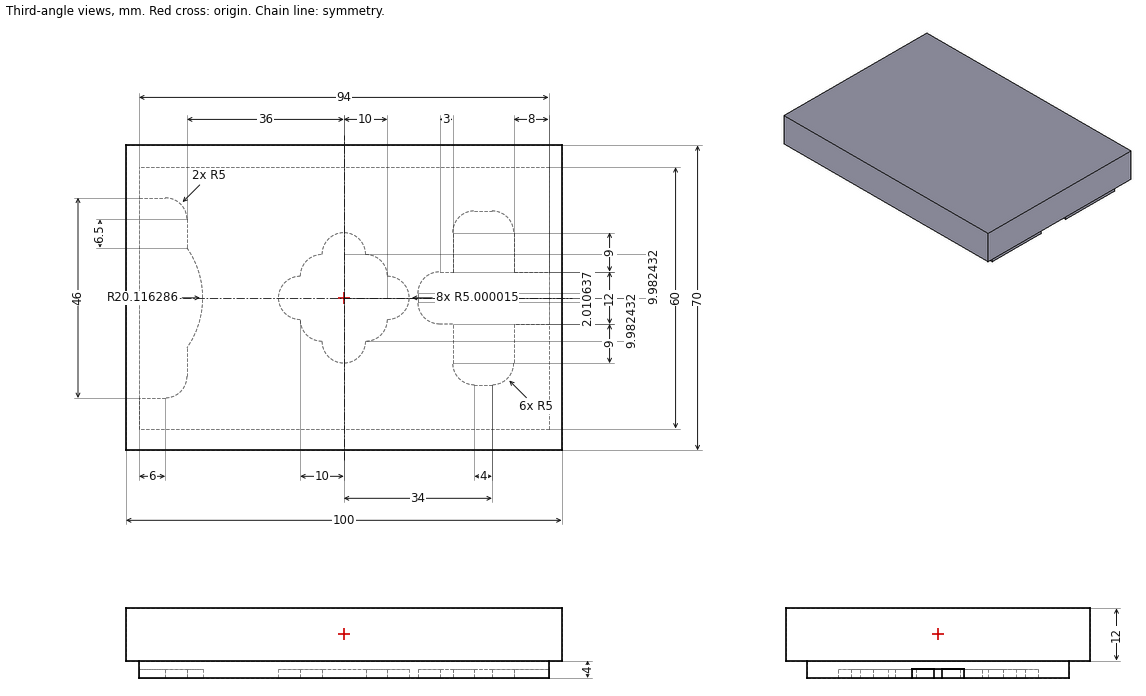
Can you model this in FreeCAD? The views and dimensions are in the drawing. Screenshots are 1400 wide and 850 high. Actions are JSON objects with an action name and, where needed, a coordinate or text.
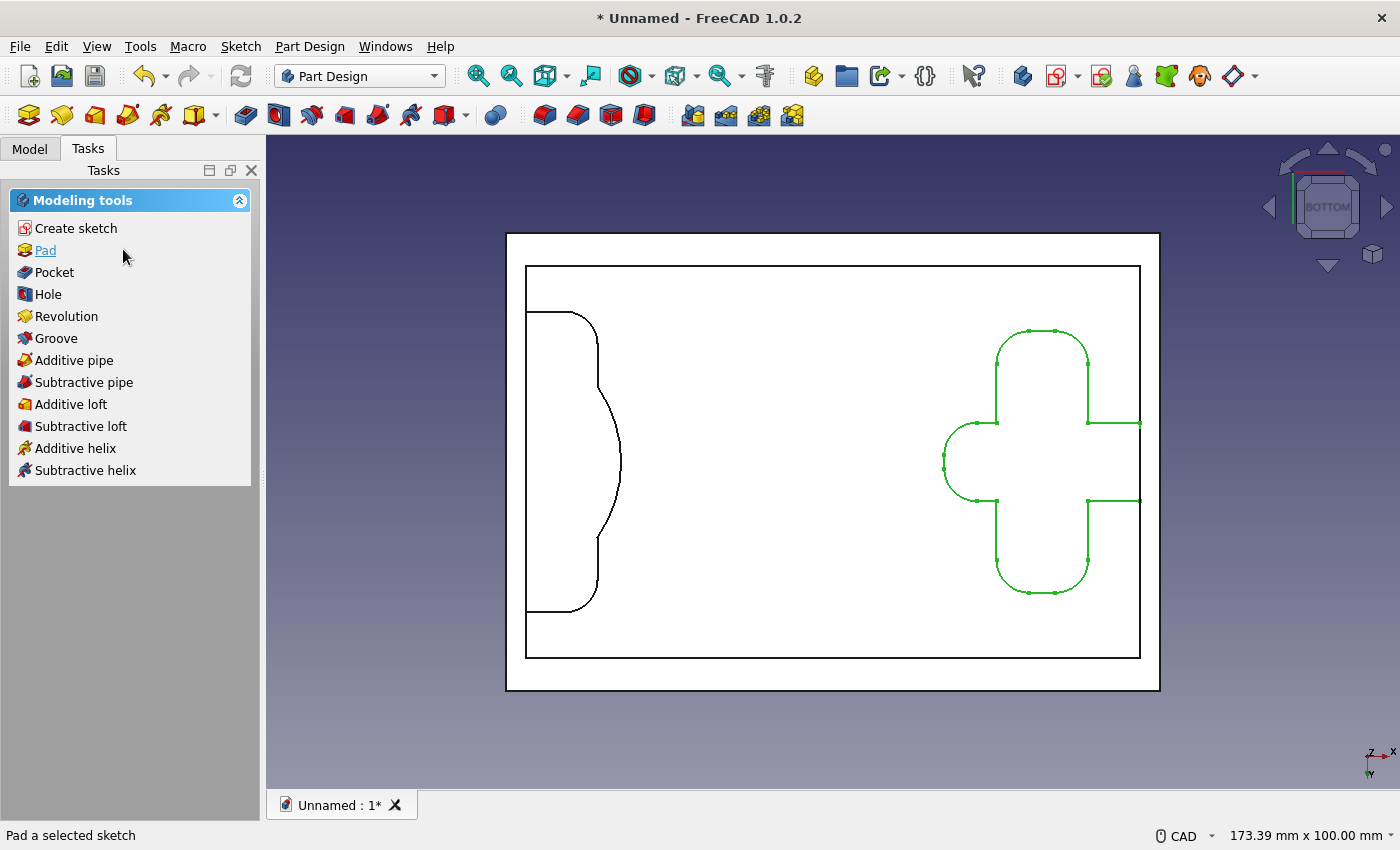
{"action": "left_click", "coordinate": [246, 116]}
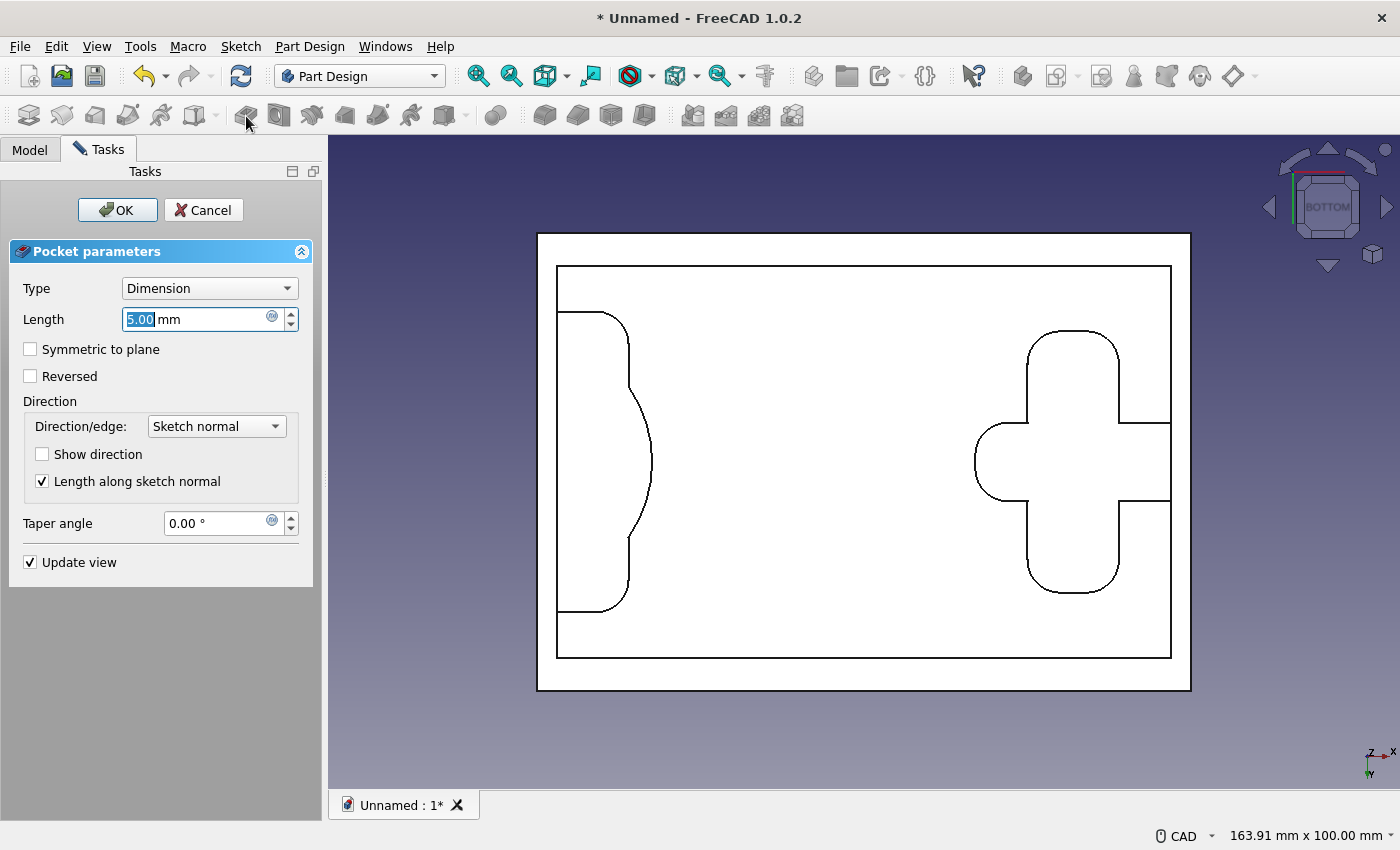
{"action": "type", "text": "4"}
{"action": "key", "text": "Tab"}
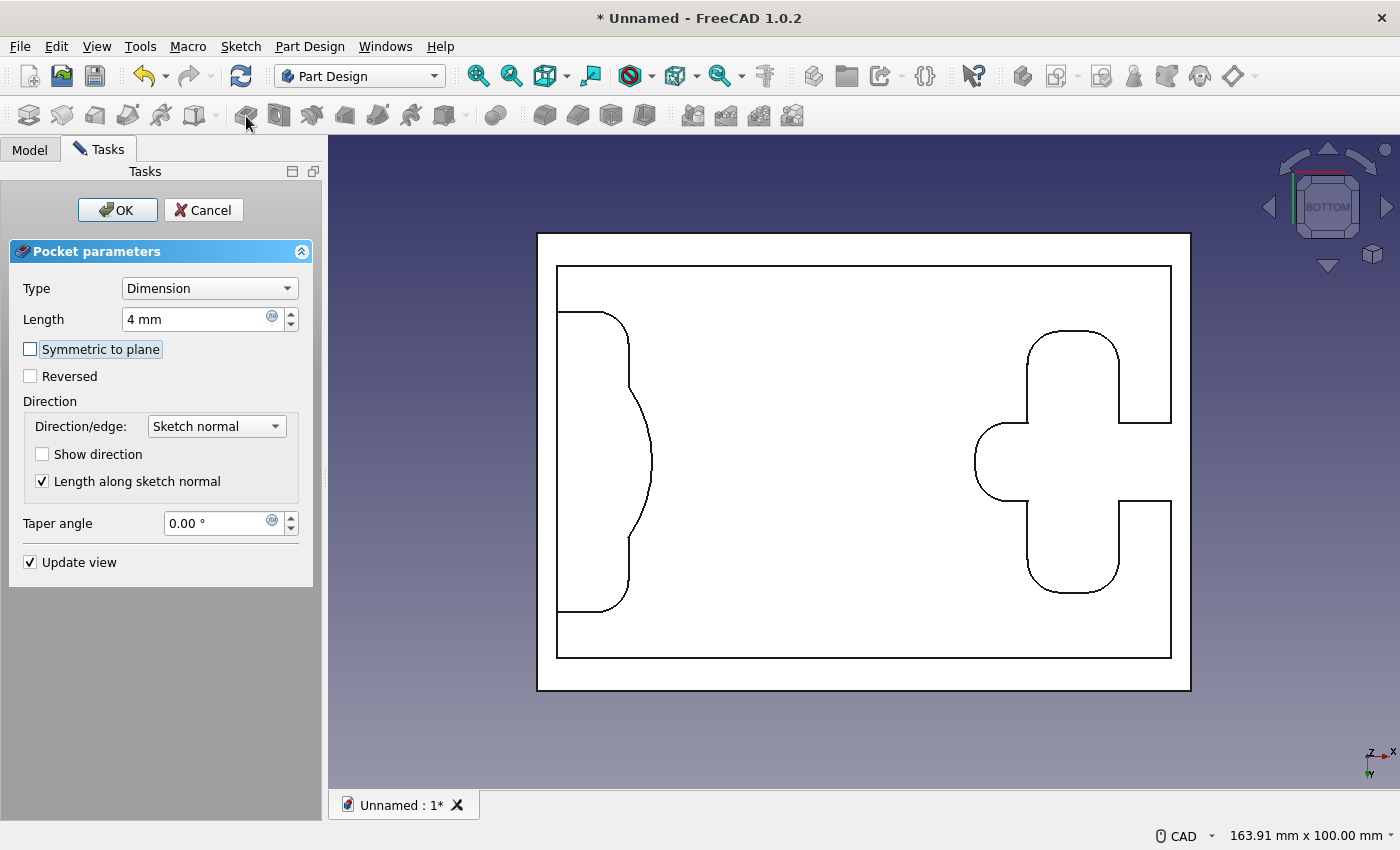
{"action": "left_click", "coordinate": [31, 349]}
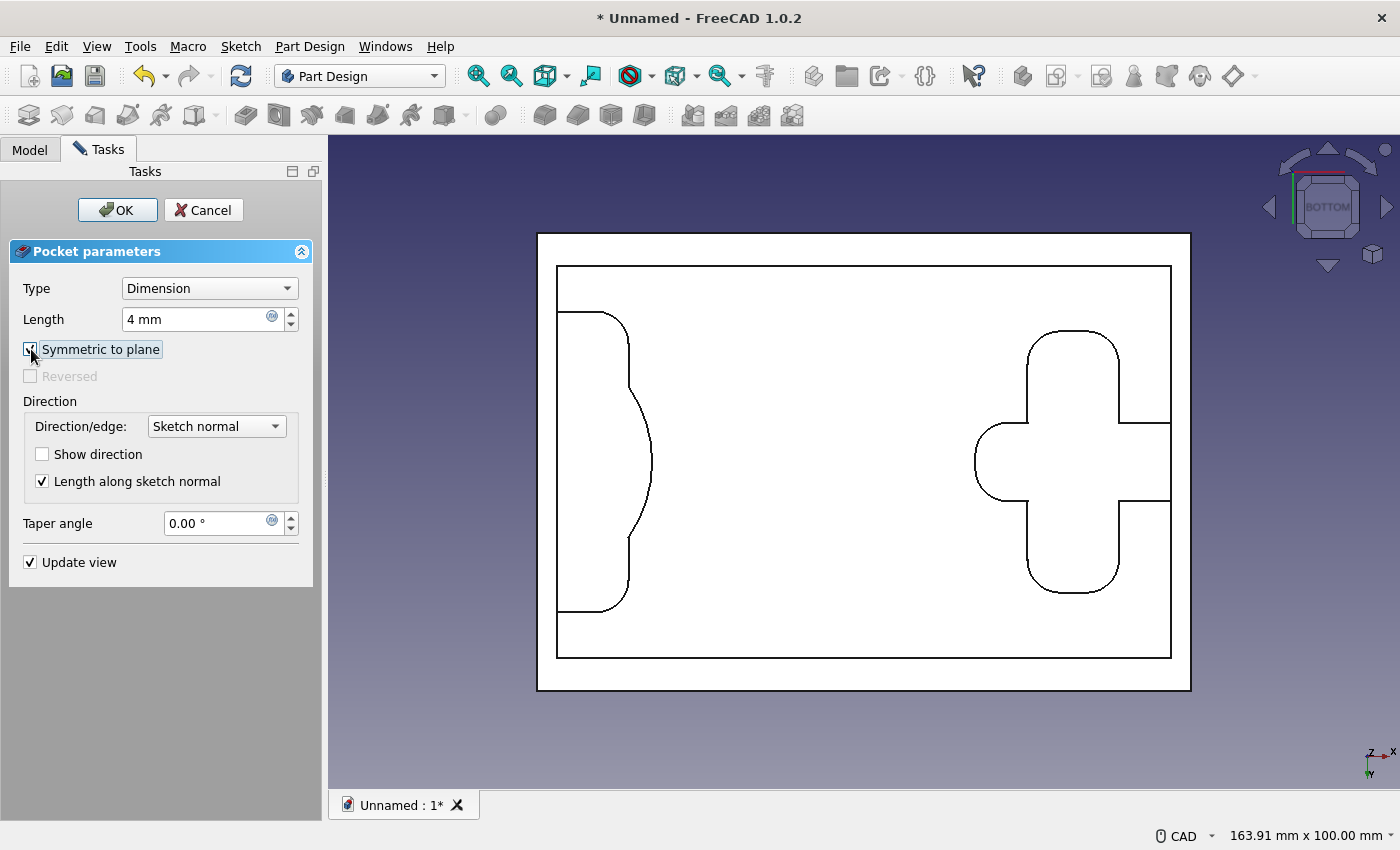
{"action": "left_click", "coordinate": [118, 210]}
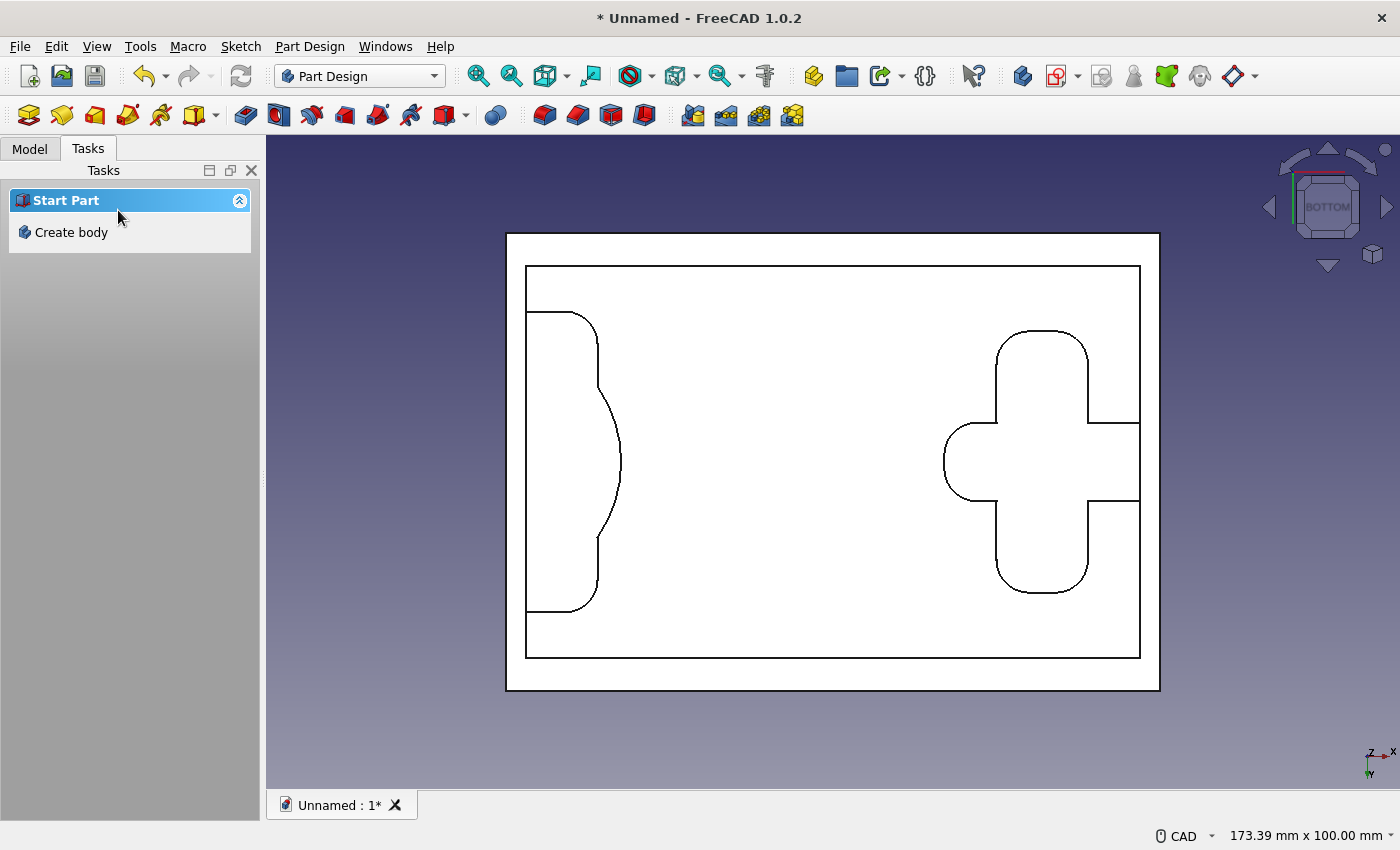
{"action": "left_click", "coordinate": [745, 405]}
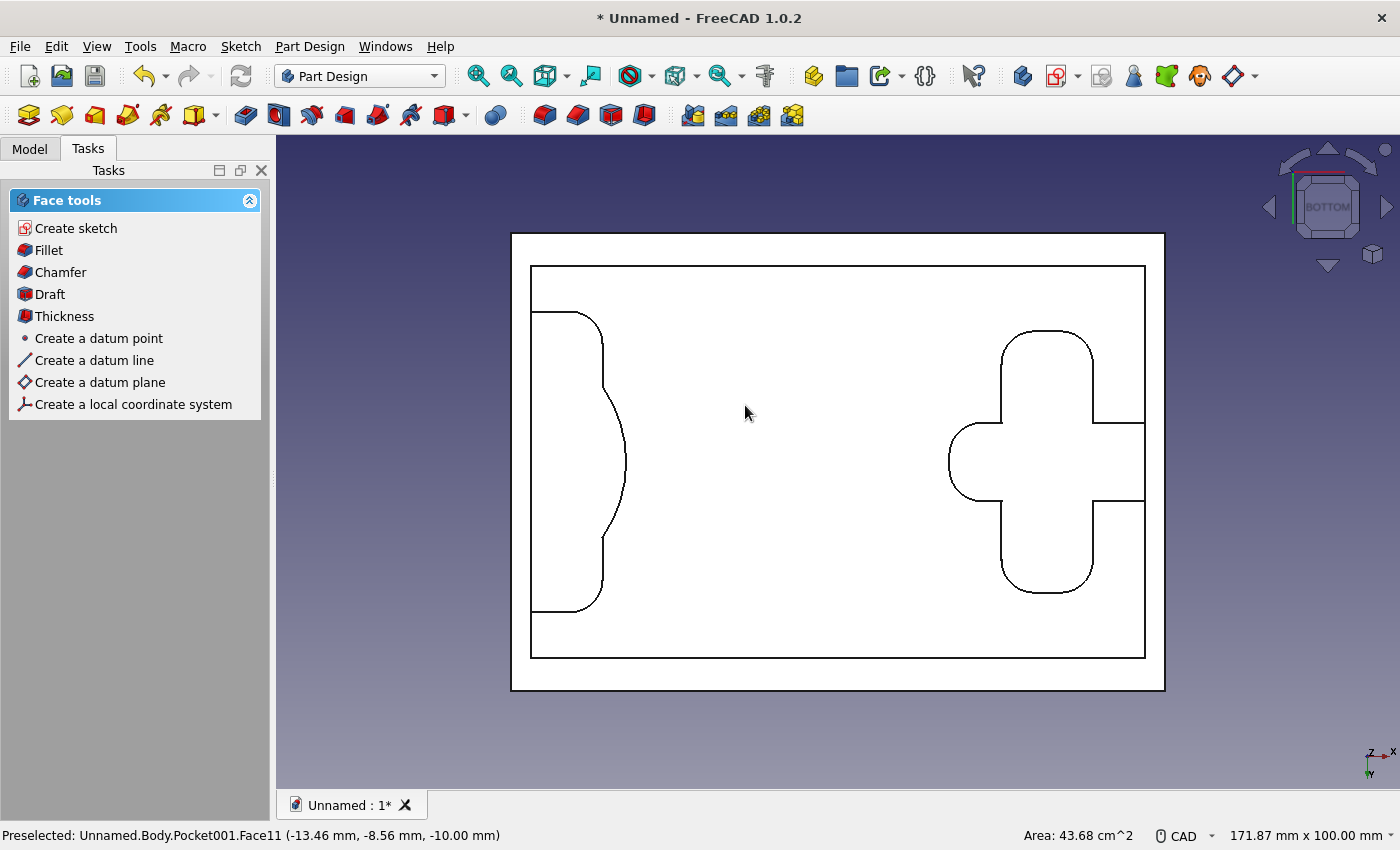
{"action": "left_click", "coordinate": [1056, 76]}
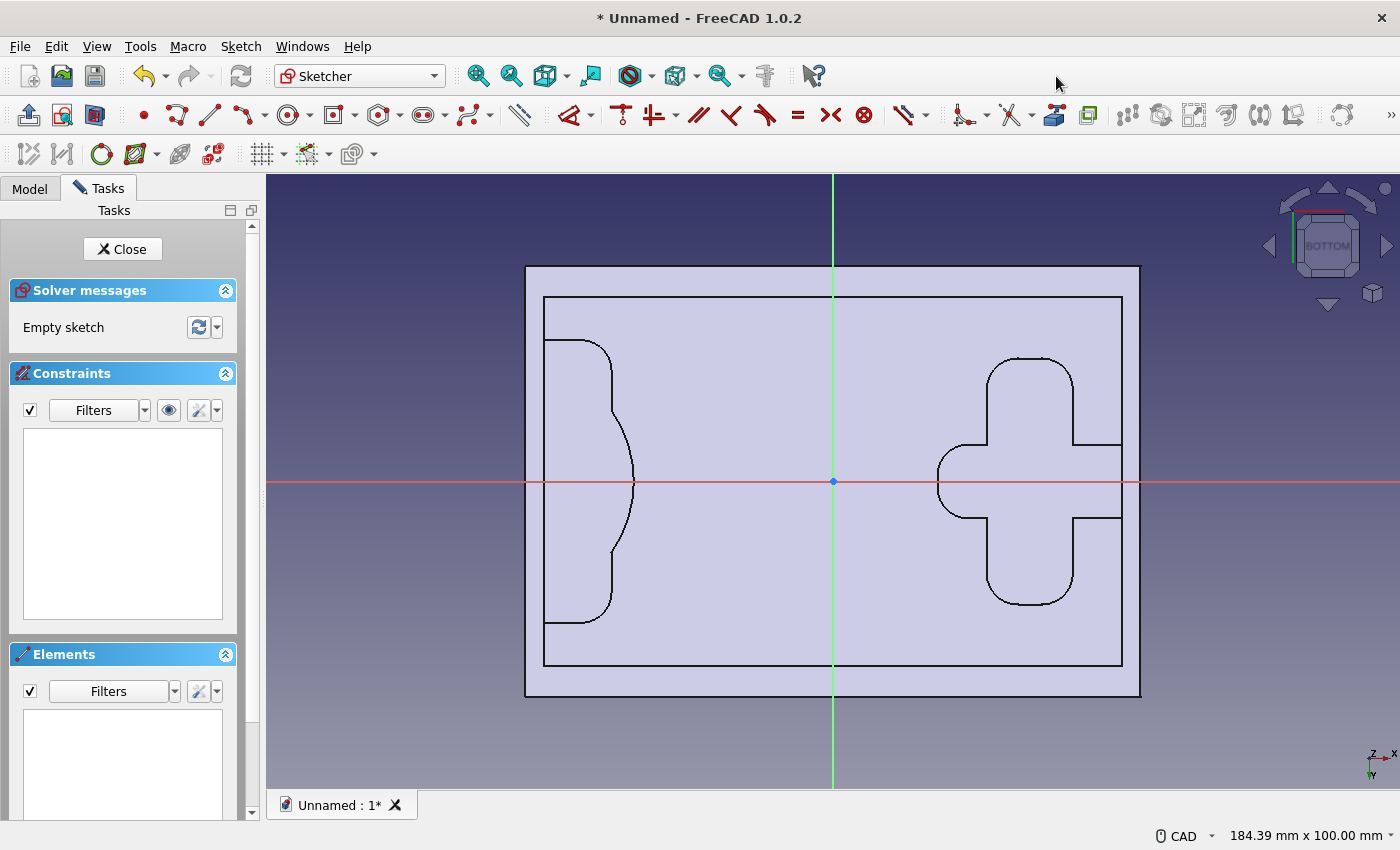
{"action": "scroll", "coordinate": [889, 482], "scroll_direction": "up", "scroll_amount": 4}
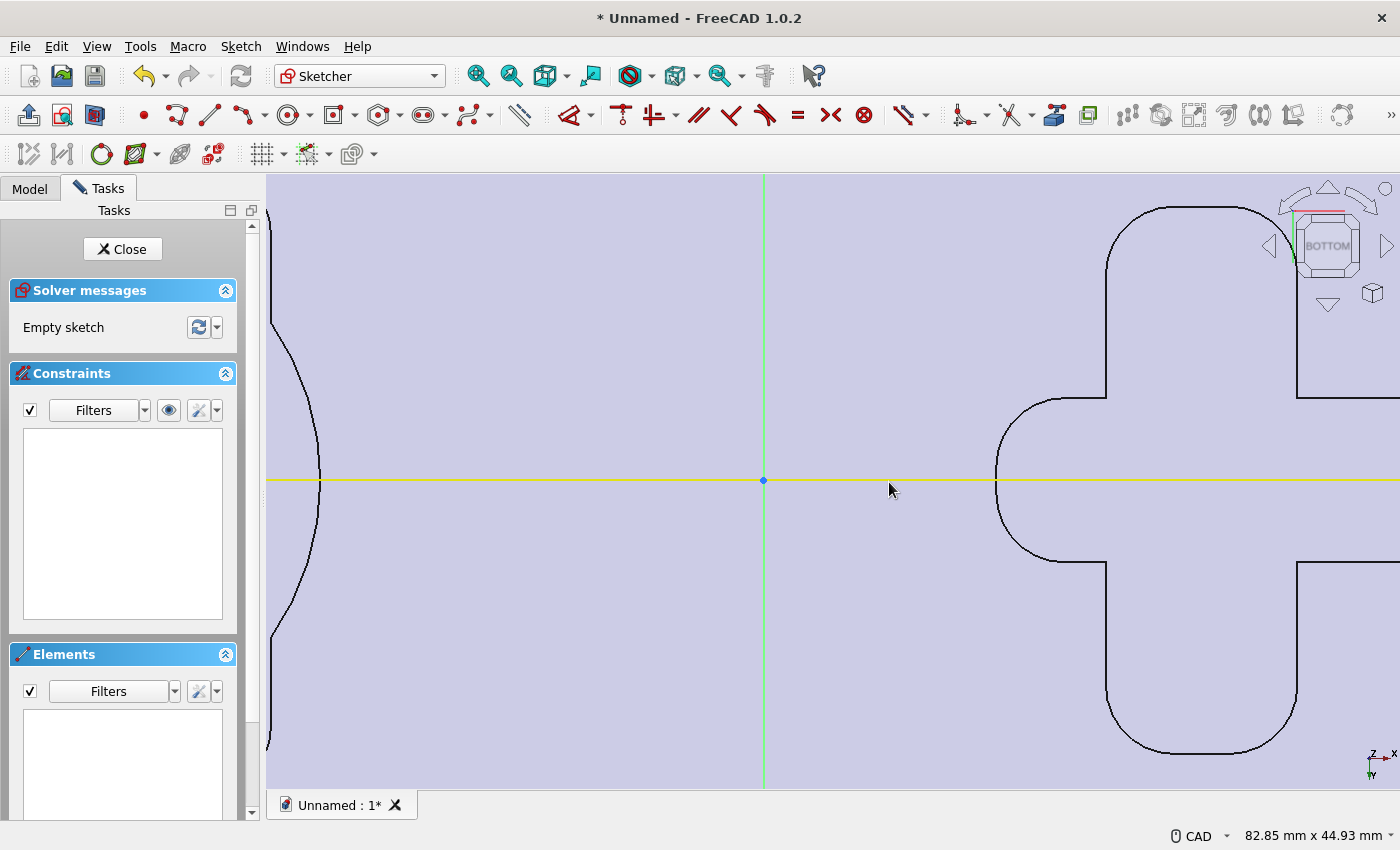
{"action": "left_click", "coordinate": [242, 116]}